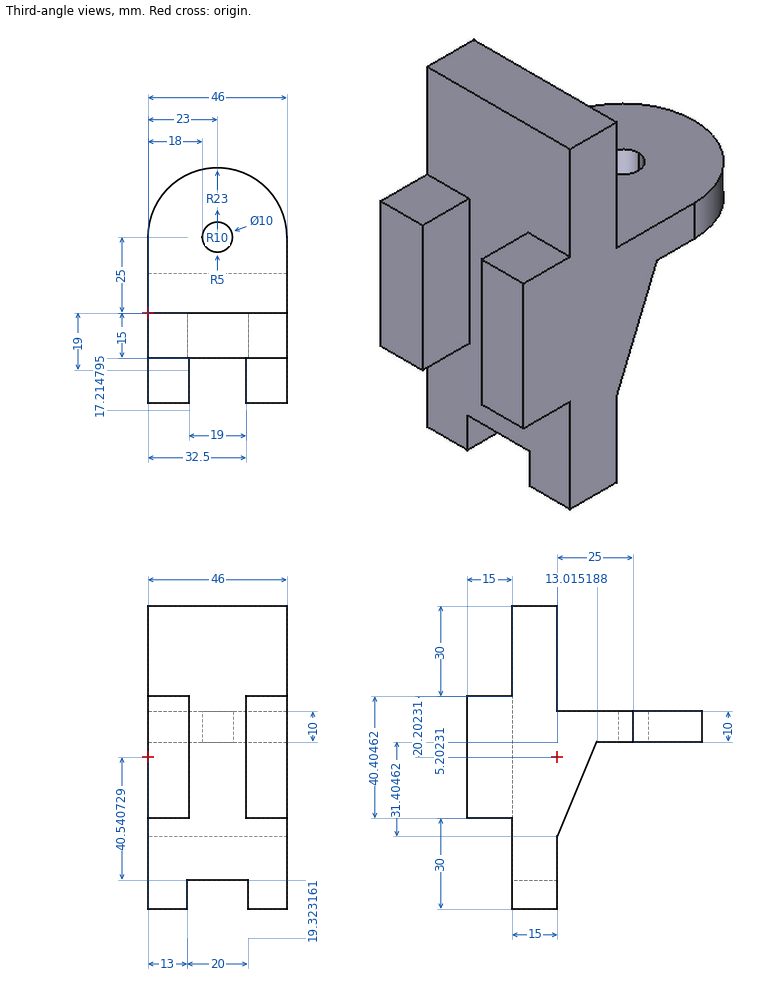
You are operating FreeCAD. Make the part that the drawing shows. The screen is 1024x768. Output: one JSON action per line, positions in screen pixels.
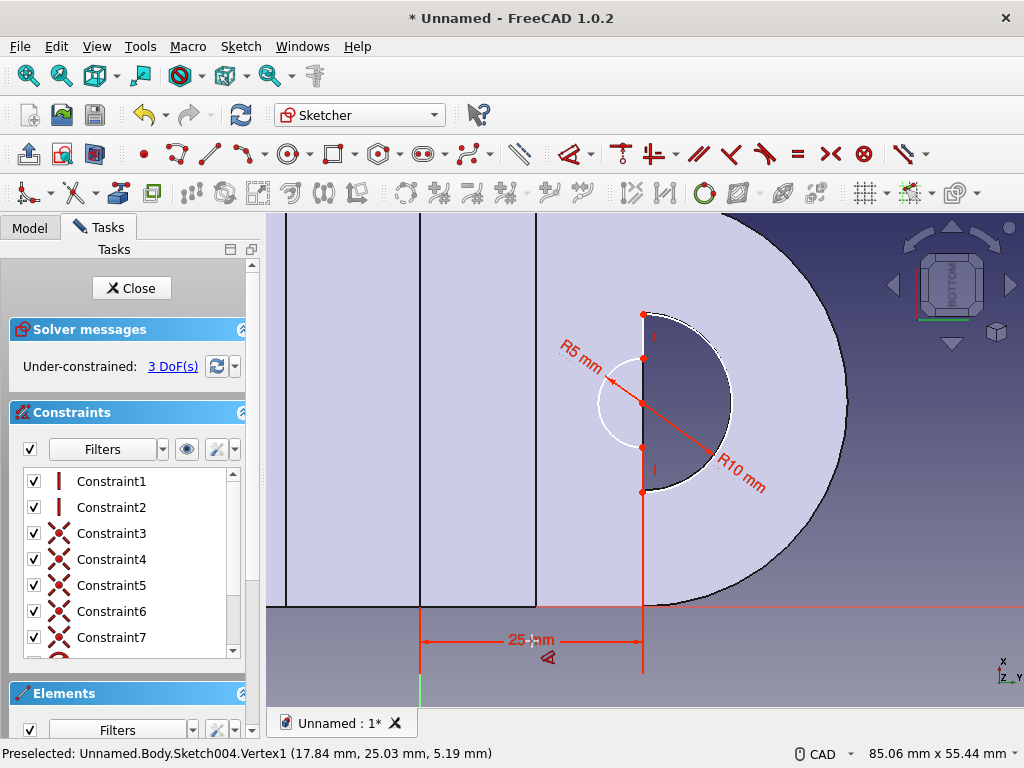
{"action": "left_click", "coordinate": [643, 448]}
{"action": "left_click", "coordinate": [386, 527]}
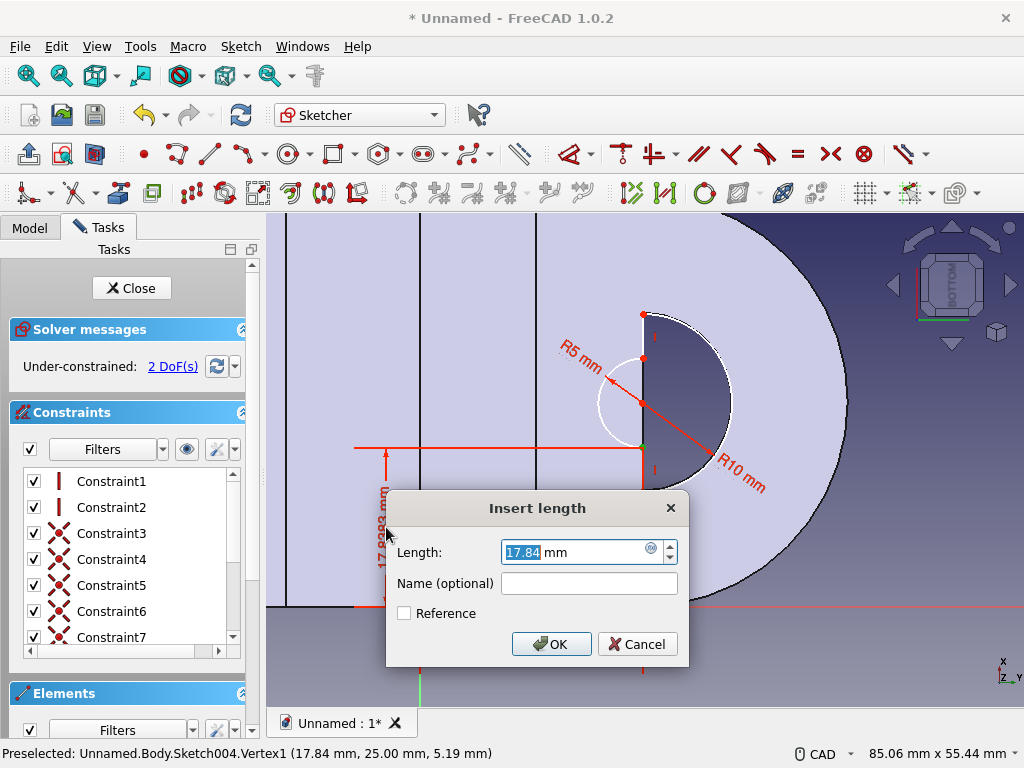
{"action": "type", "text": "18"}
{"action": "key", "text": "Return"}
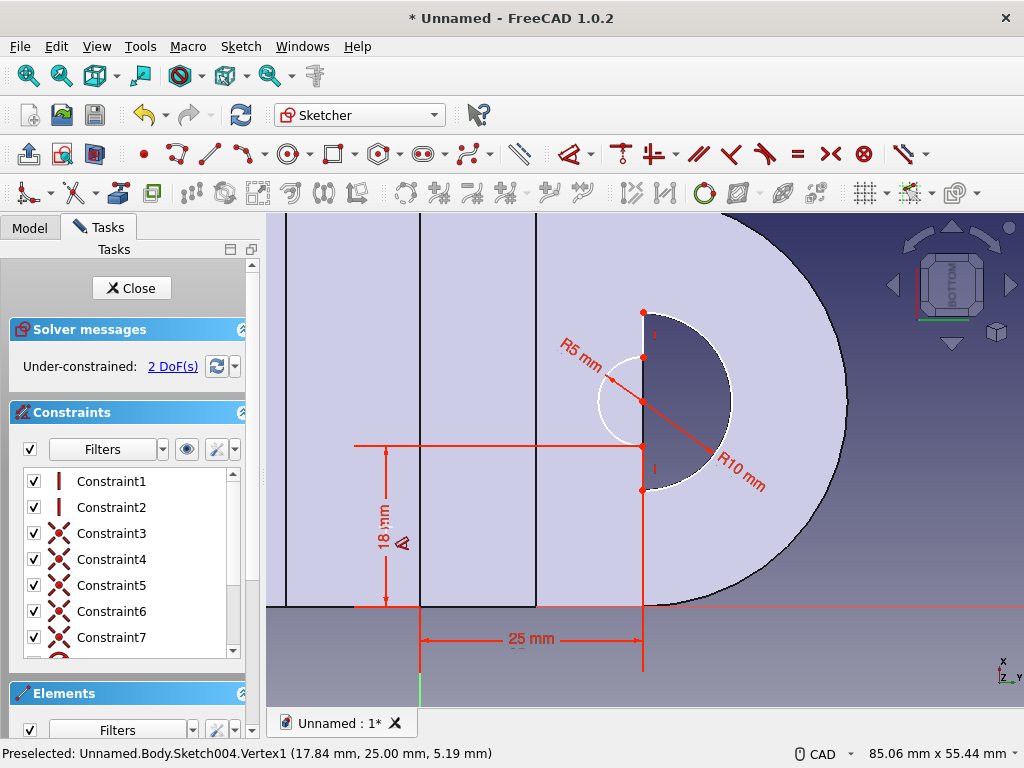
{"action": "left_click", "coordinate": [643, 313]}
{"action": "left_click", "coordinate": [453, 641]}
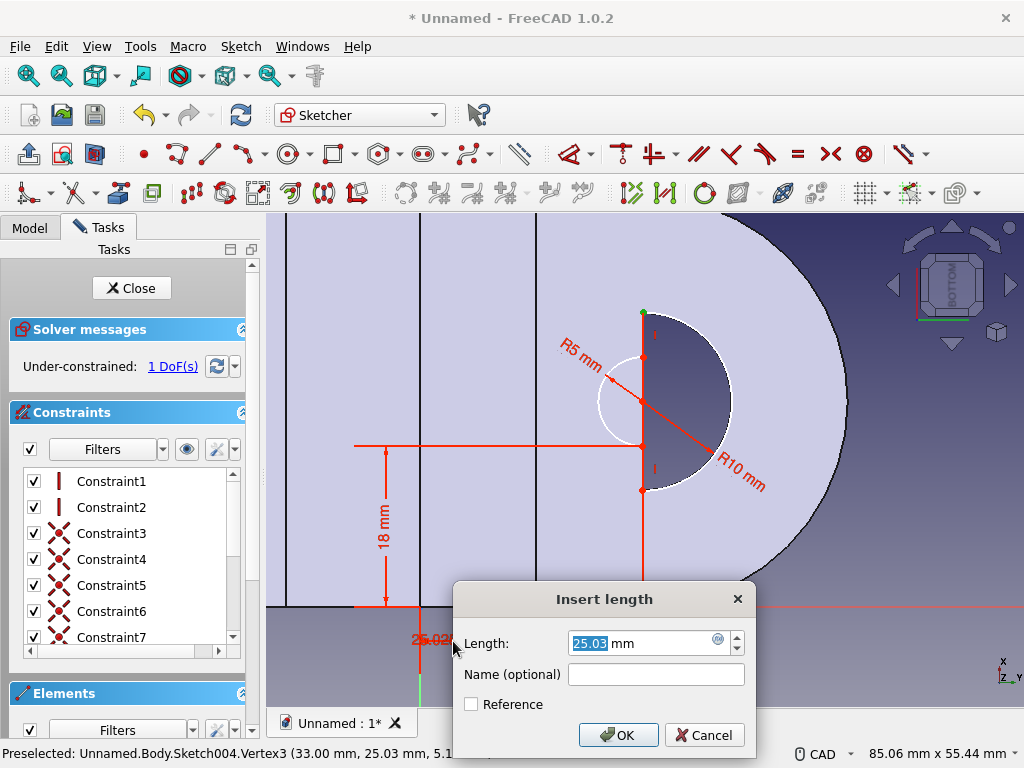
{"action": "type", "text": "25"}
{"action": "key", "text": "Return"}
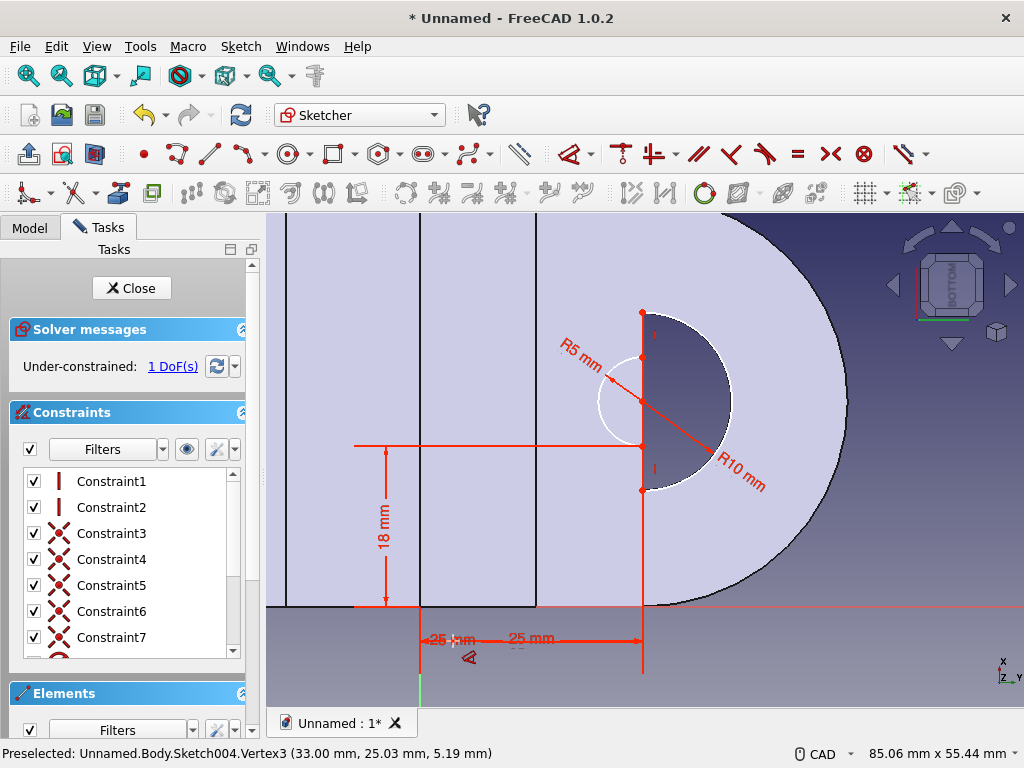
{"action": "left_click", "coordinate": [643, 402]}
{"action": "left_click", "coordinate": [610, 641]}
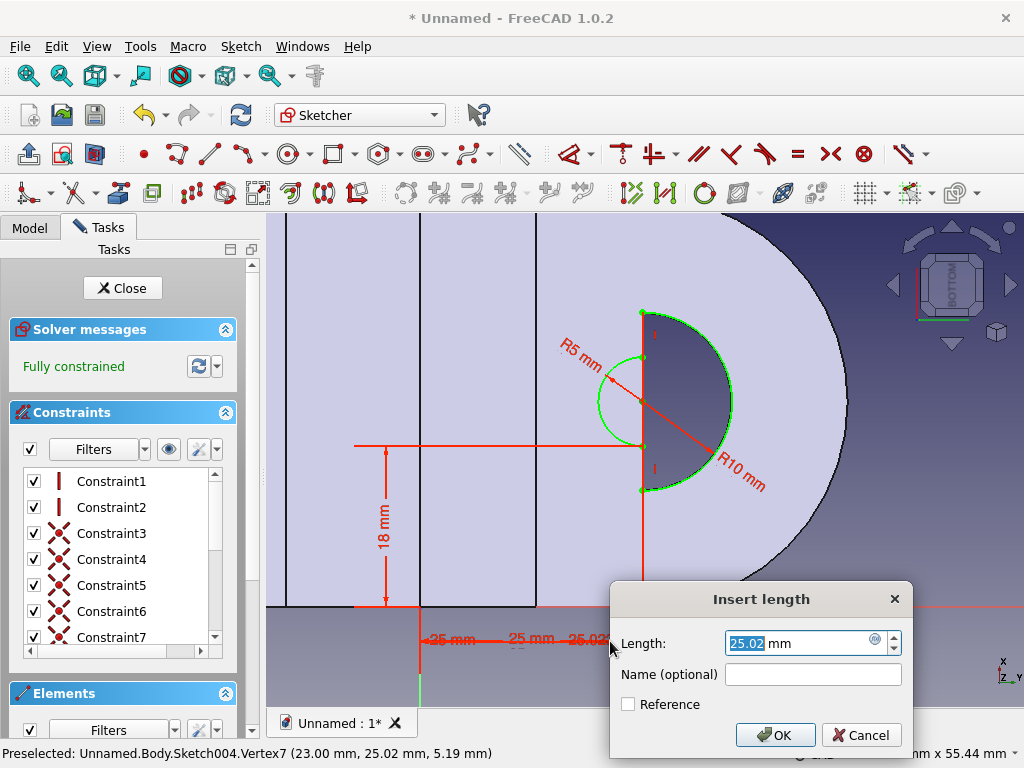
{"action": "type", "text": "25"}
{"action": "key", "text": "Return"}
{"action": "key", "text": "Escape"}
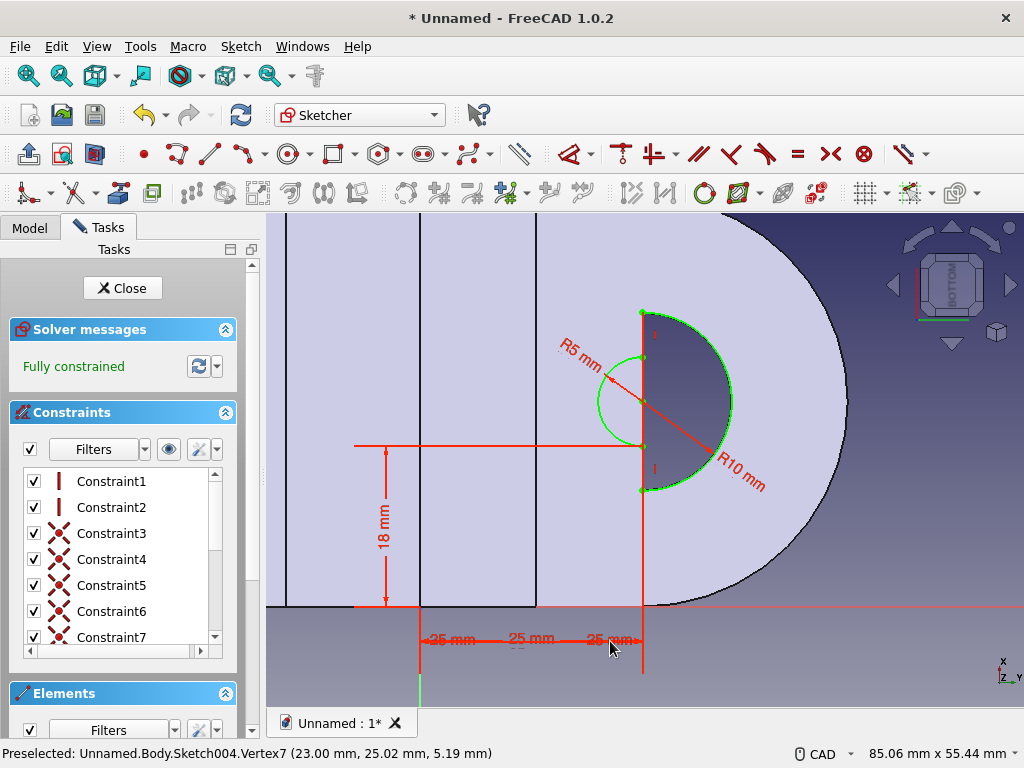
{"action": "left_click", "coordinate": [123, 288]}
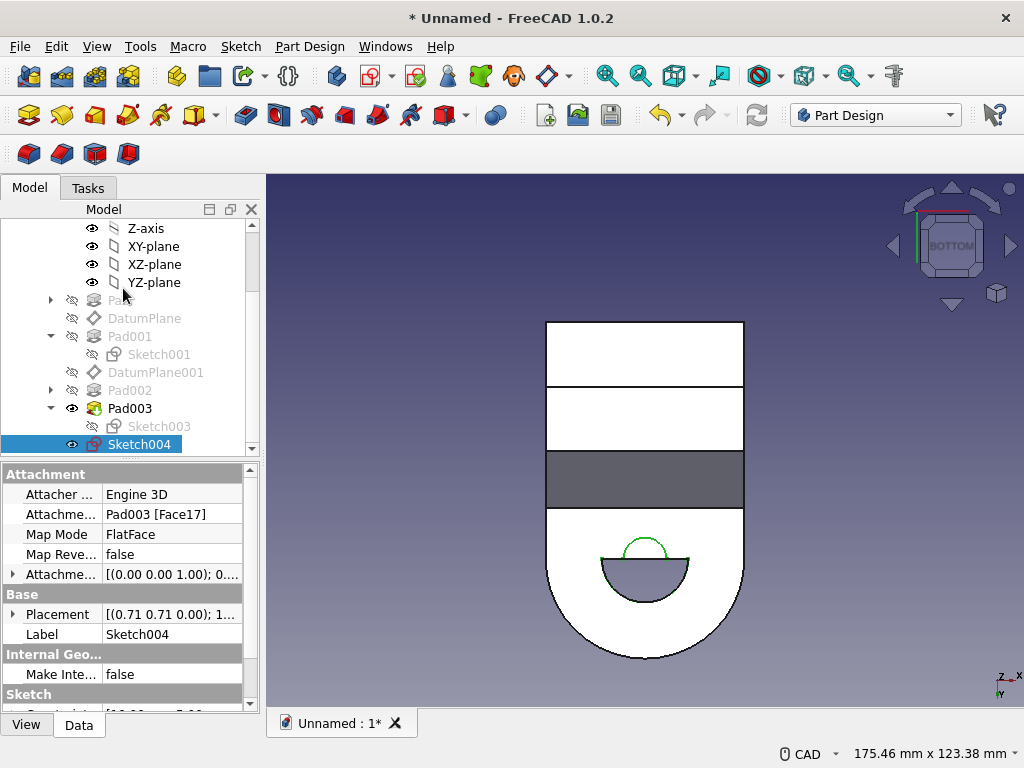
{"action": "left_click", "coordinate": [29, 116]}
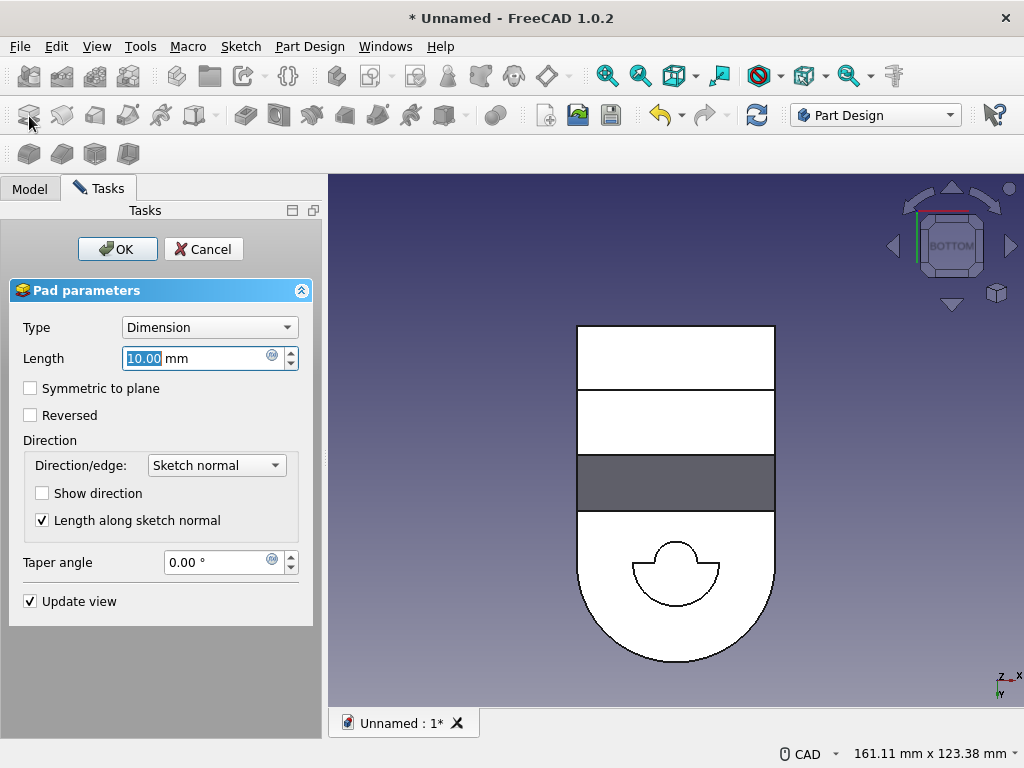
{"action": "type", "text": "10"}
{"action": "key", "text": "Tab"}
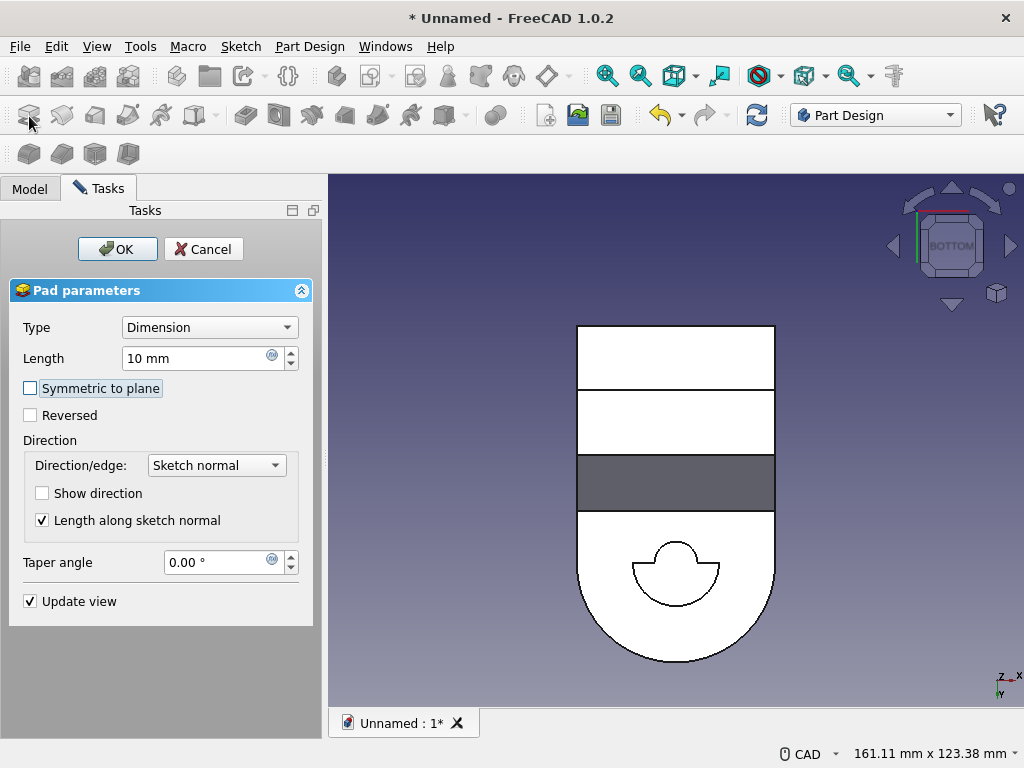
{"action": "left_click", "coordinate": [31, 415]}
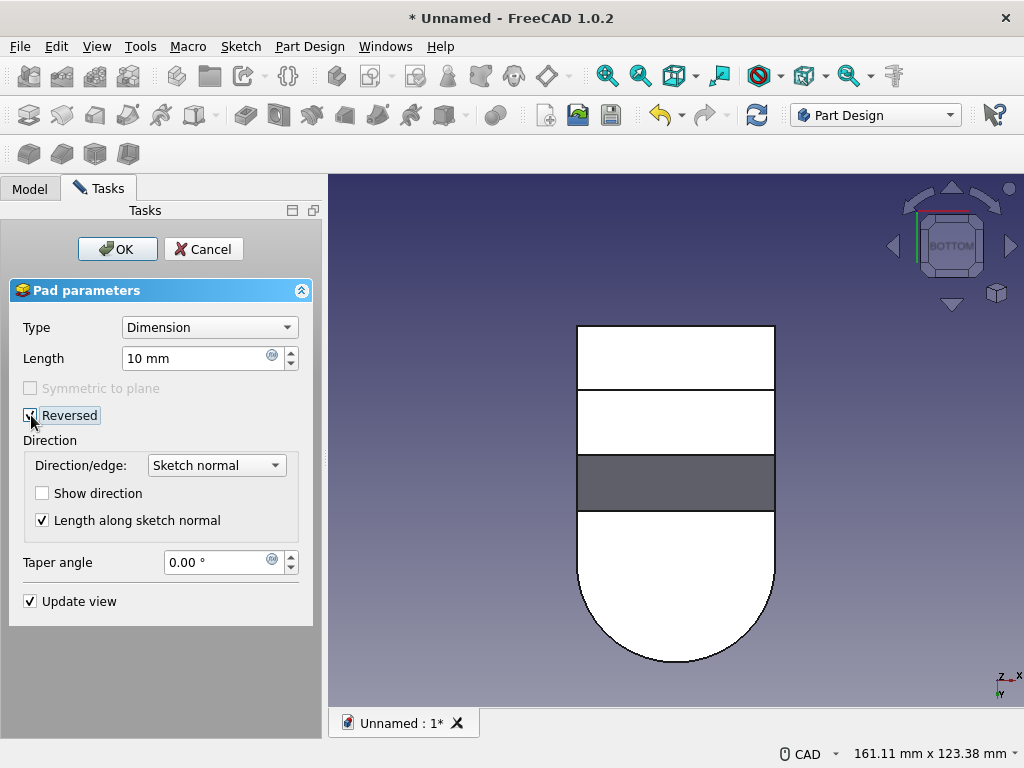
{"action": "left_click", "coordinate": [118, 249]}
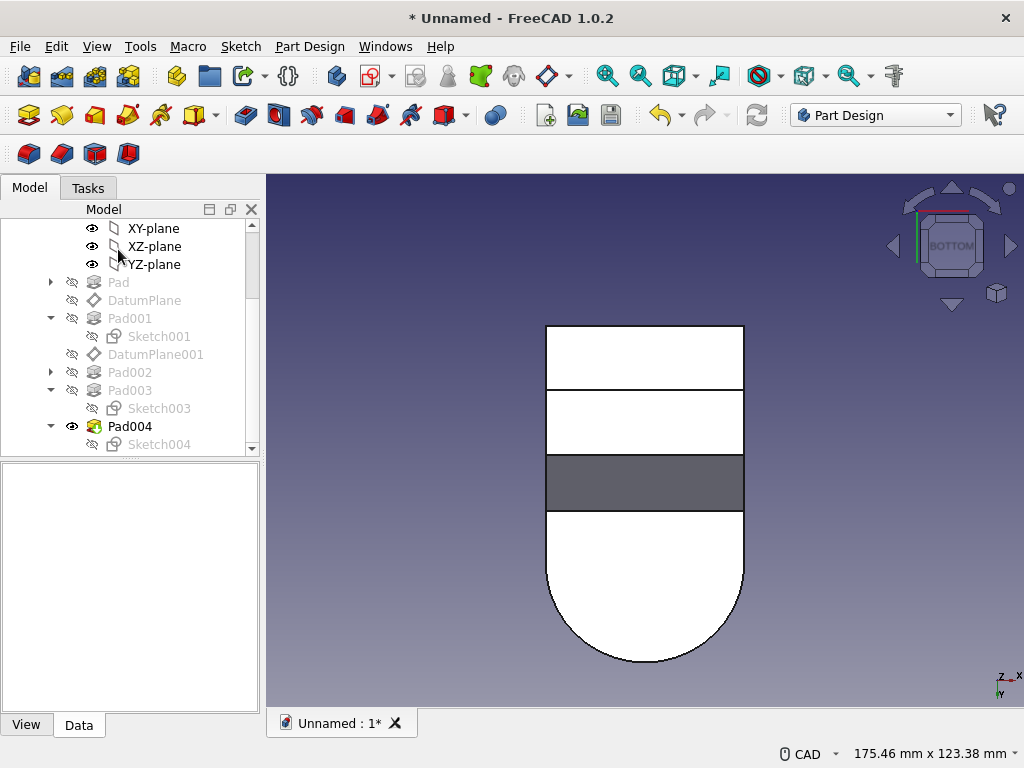
{"action": "left_click", "coordinate": [645, 586]}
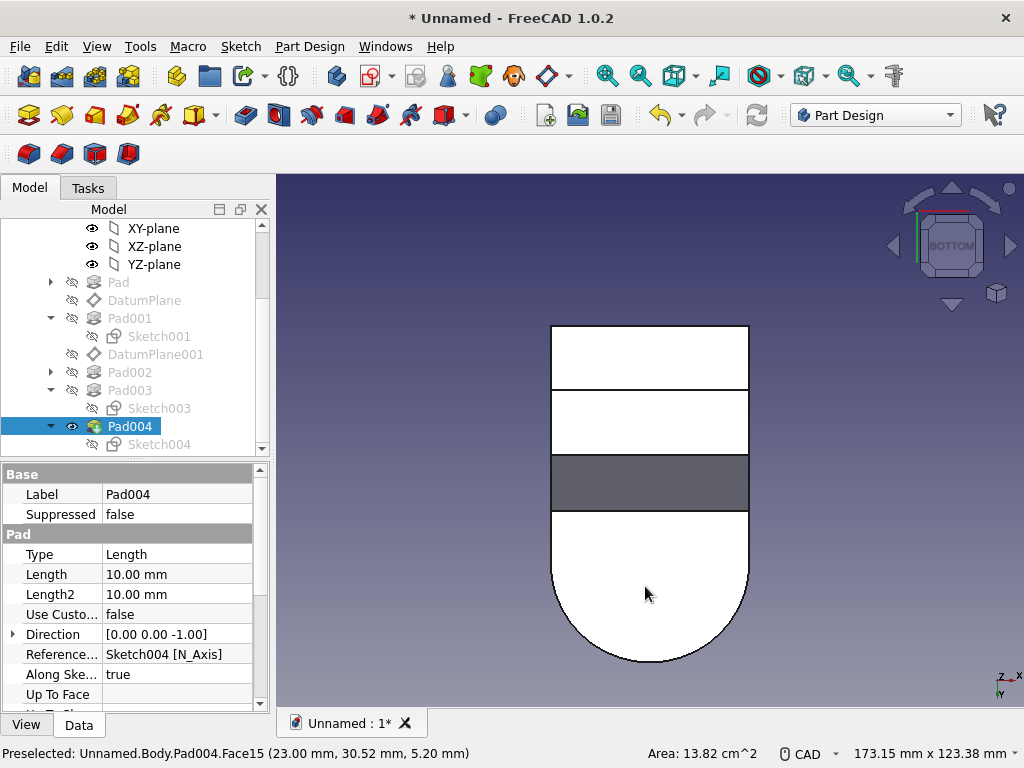
{"action": "left_click", "coordinate": [370, 76]}